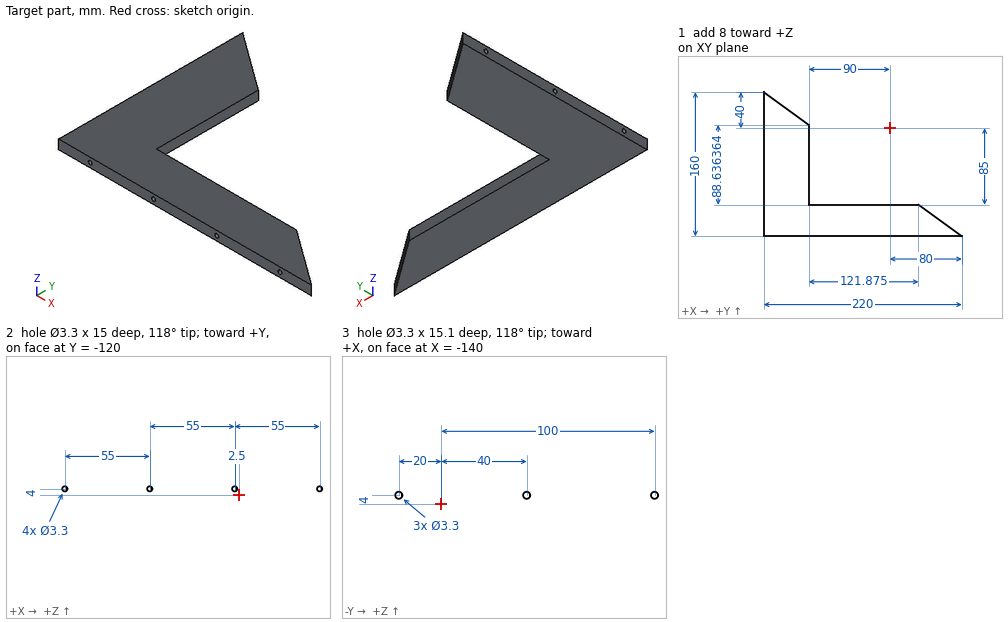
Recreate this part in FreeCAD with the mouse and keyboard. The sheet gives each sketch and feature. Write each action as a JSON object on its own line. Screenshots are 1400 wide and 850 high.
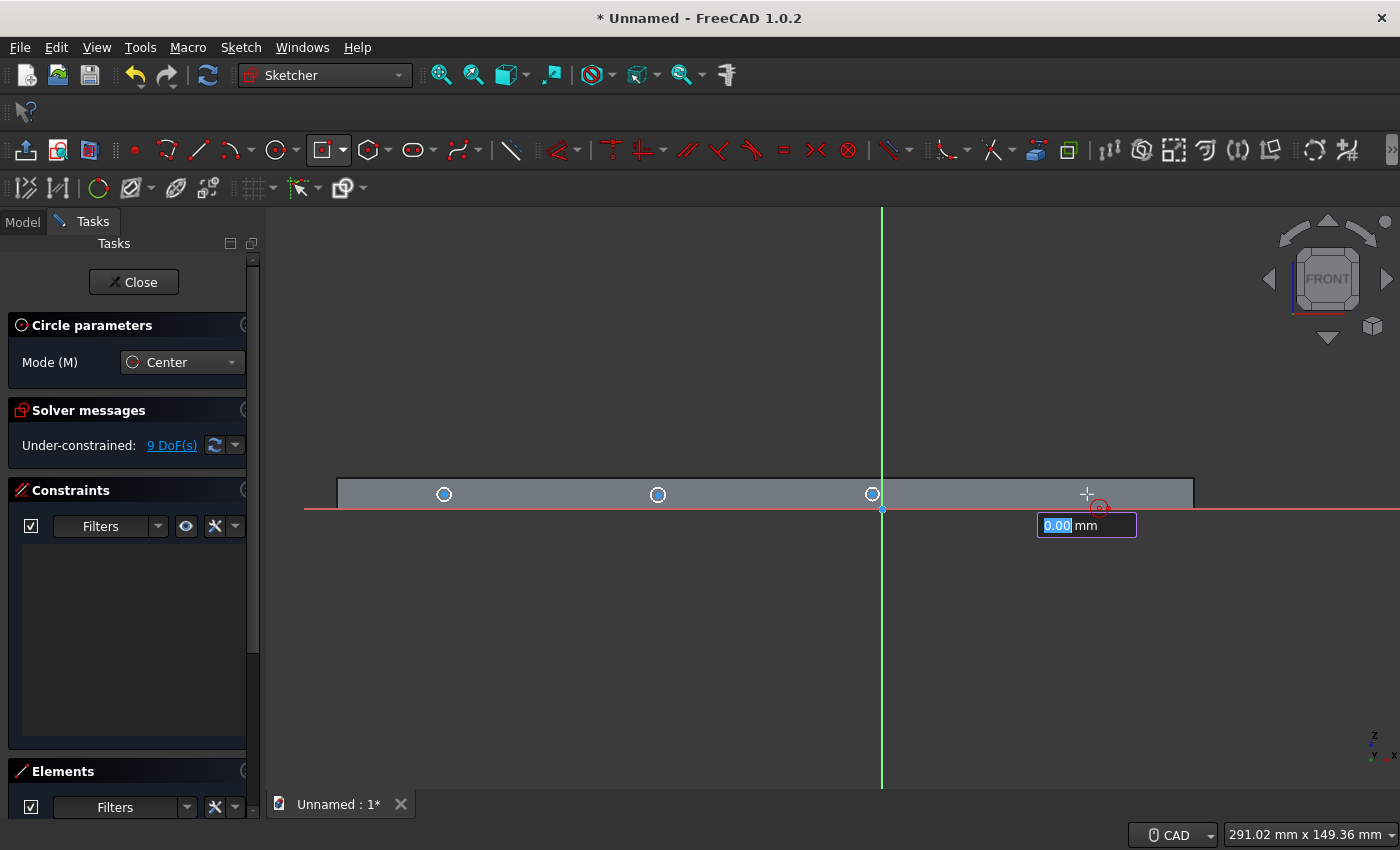
{"action": "scroll", "coordinate": [1091, 489], "scroll_direction": "up", "scroll_amount": 5}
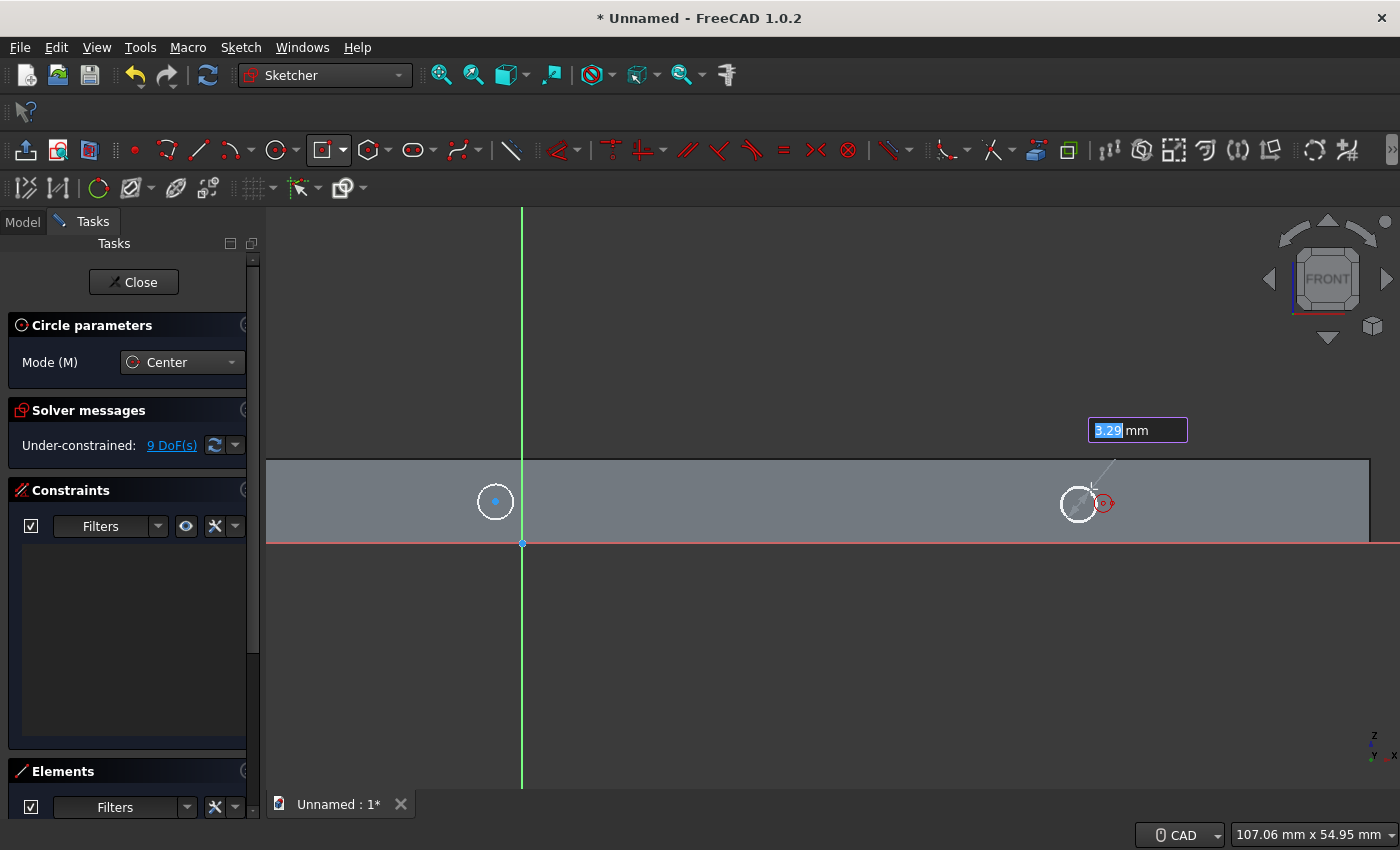
{"action": "left_click", "coordinate": [1091, 489]}
{"action": "key", "text": "Escape"}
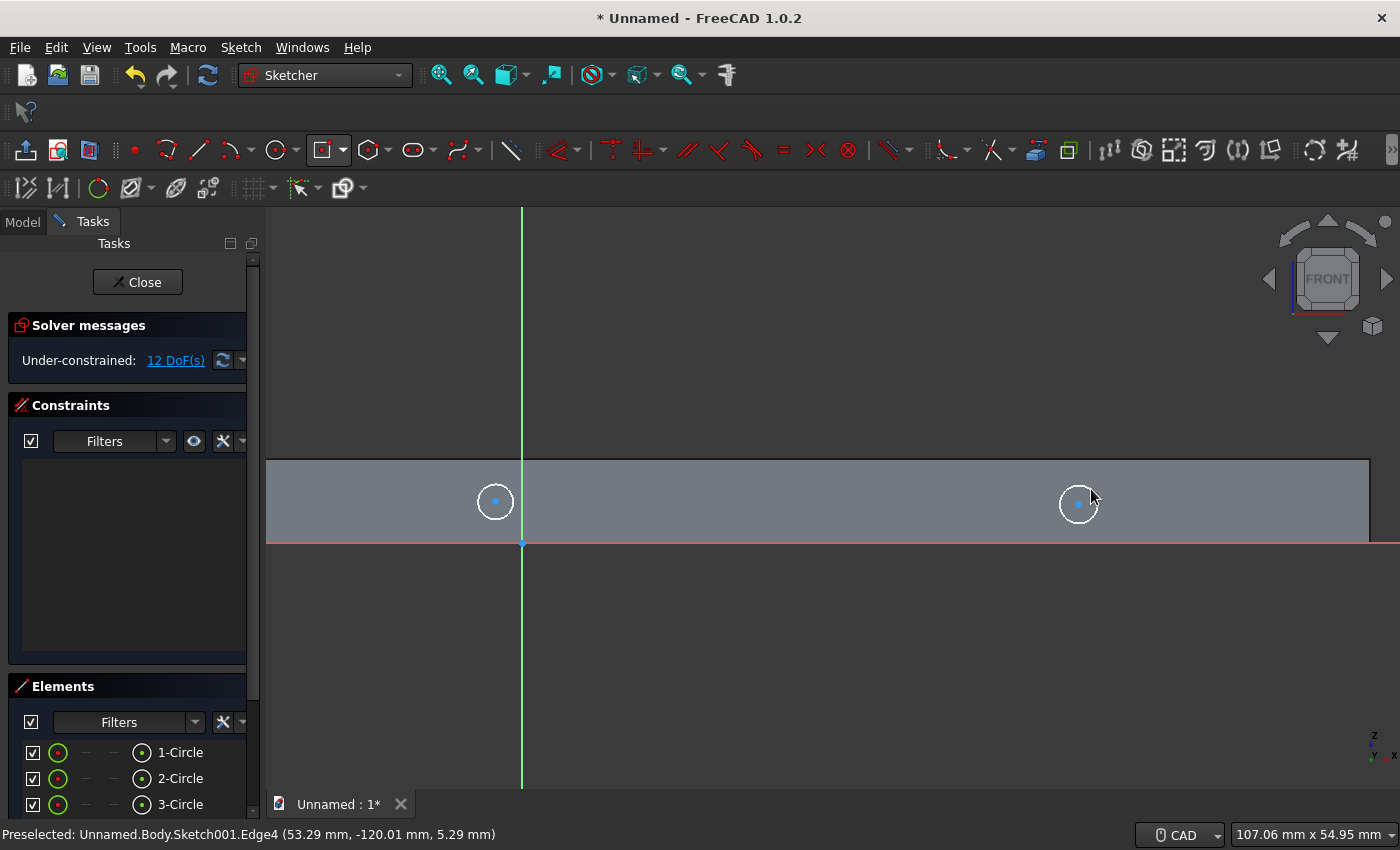
{"action": "scroll", "coordinate": [1090, 489], "scroll_direction": "down", "scroll_amount": 5}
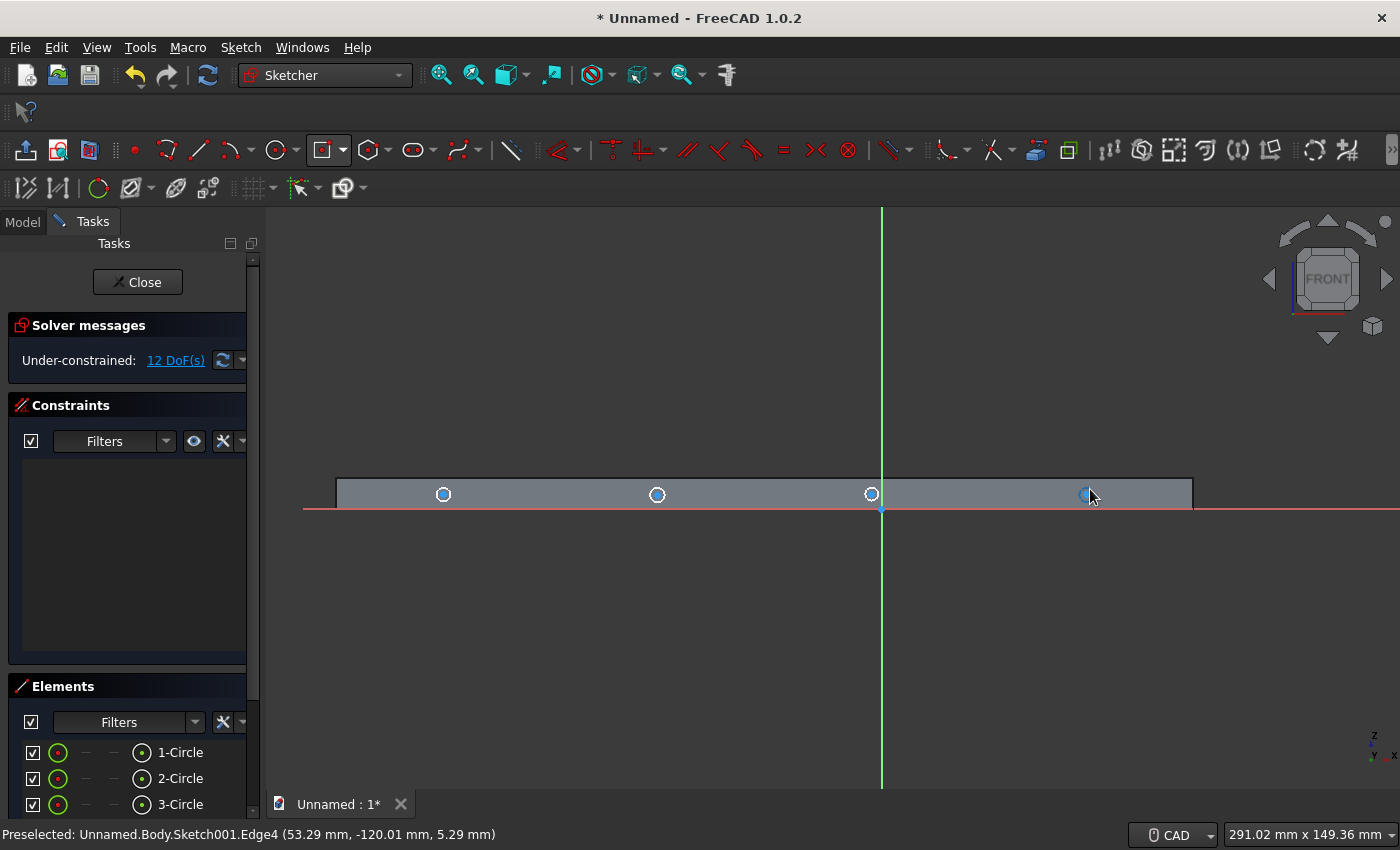
{"action": "scroll", "coordinate": [448, 490], "scroll_direction": "up", "scroll_amount": 4}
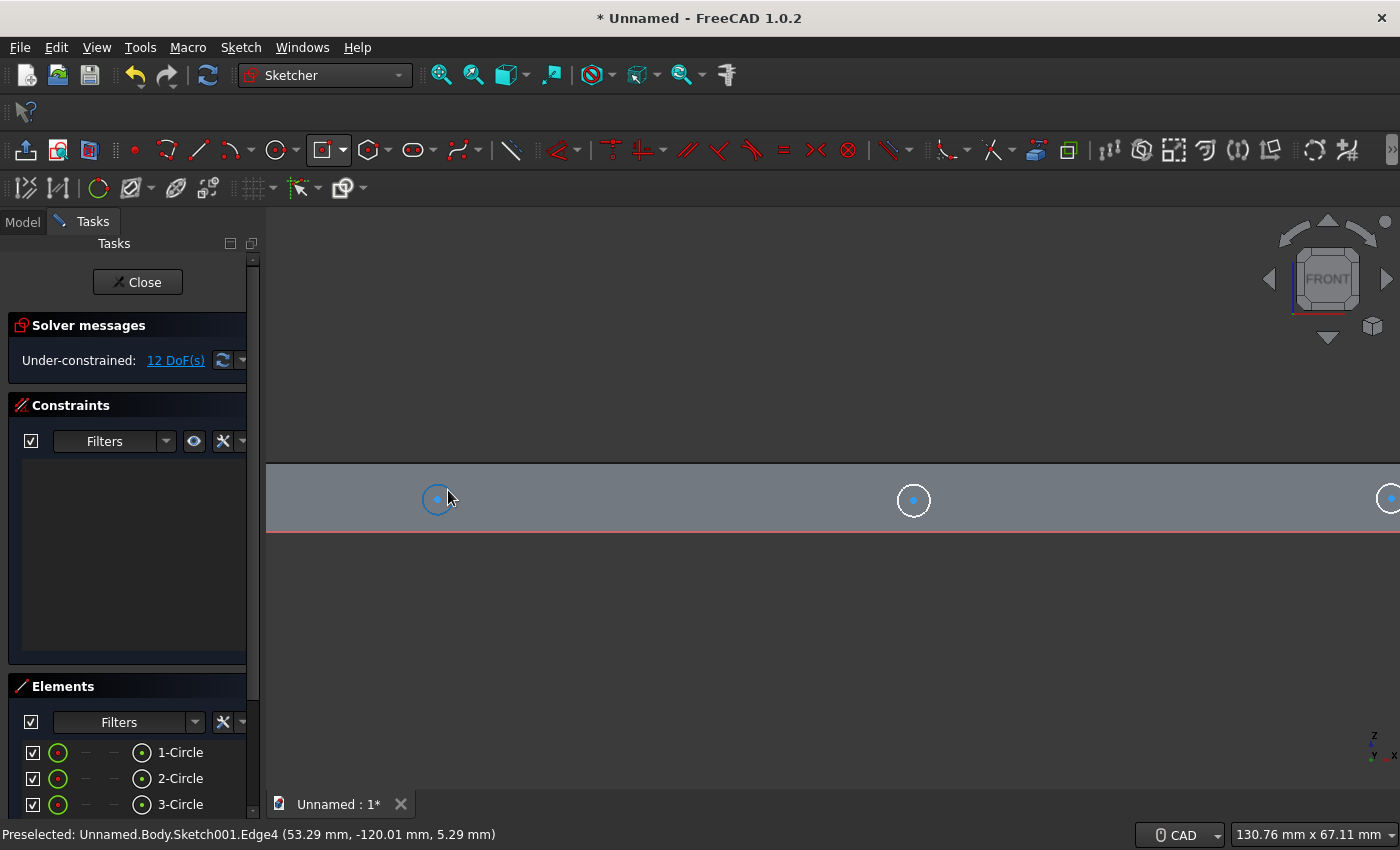
{"action": "left_click", "coordinate": [448, 489]}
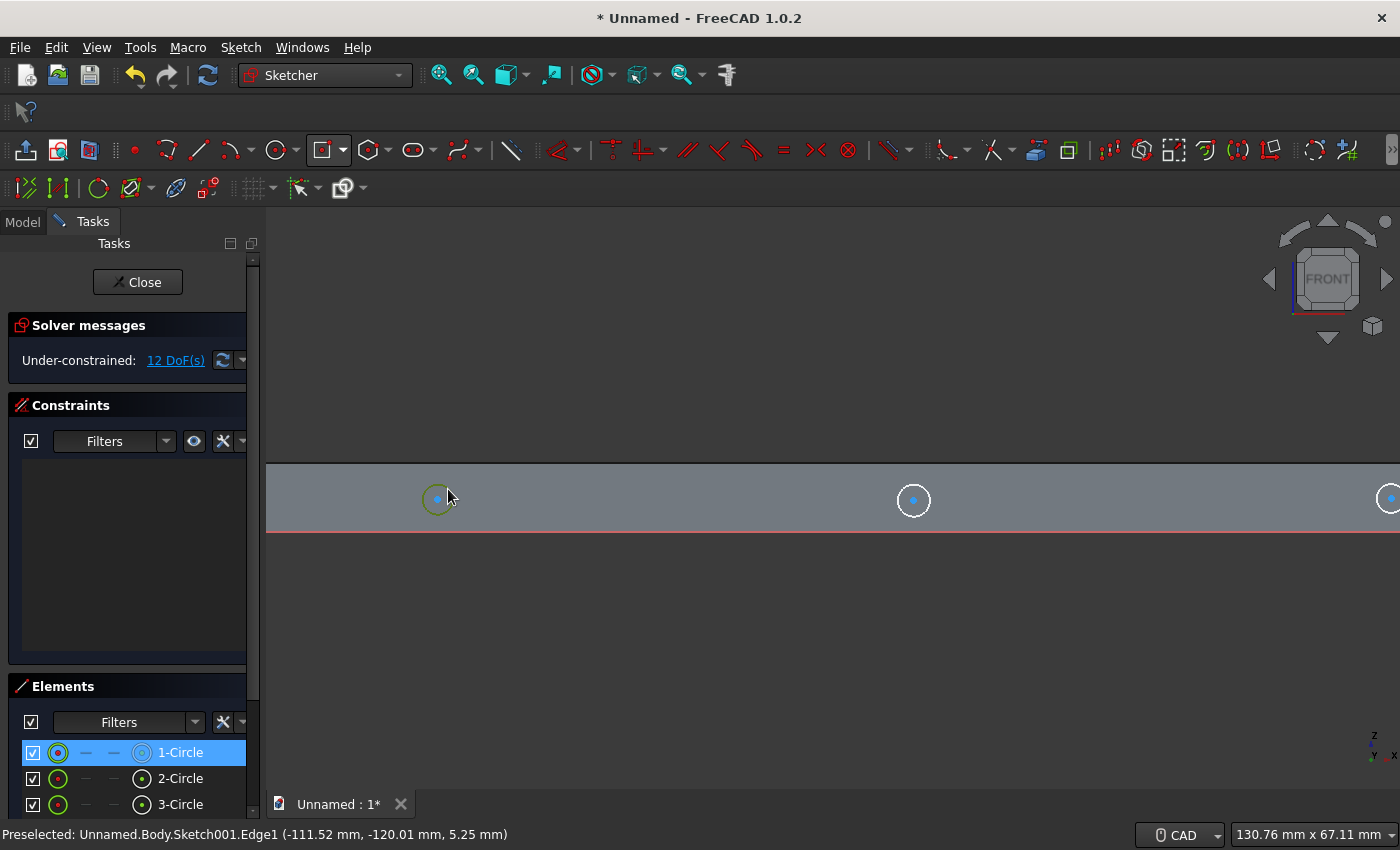
{"action": "left_click", "coordinate": [925, 489]}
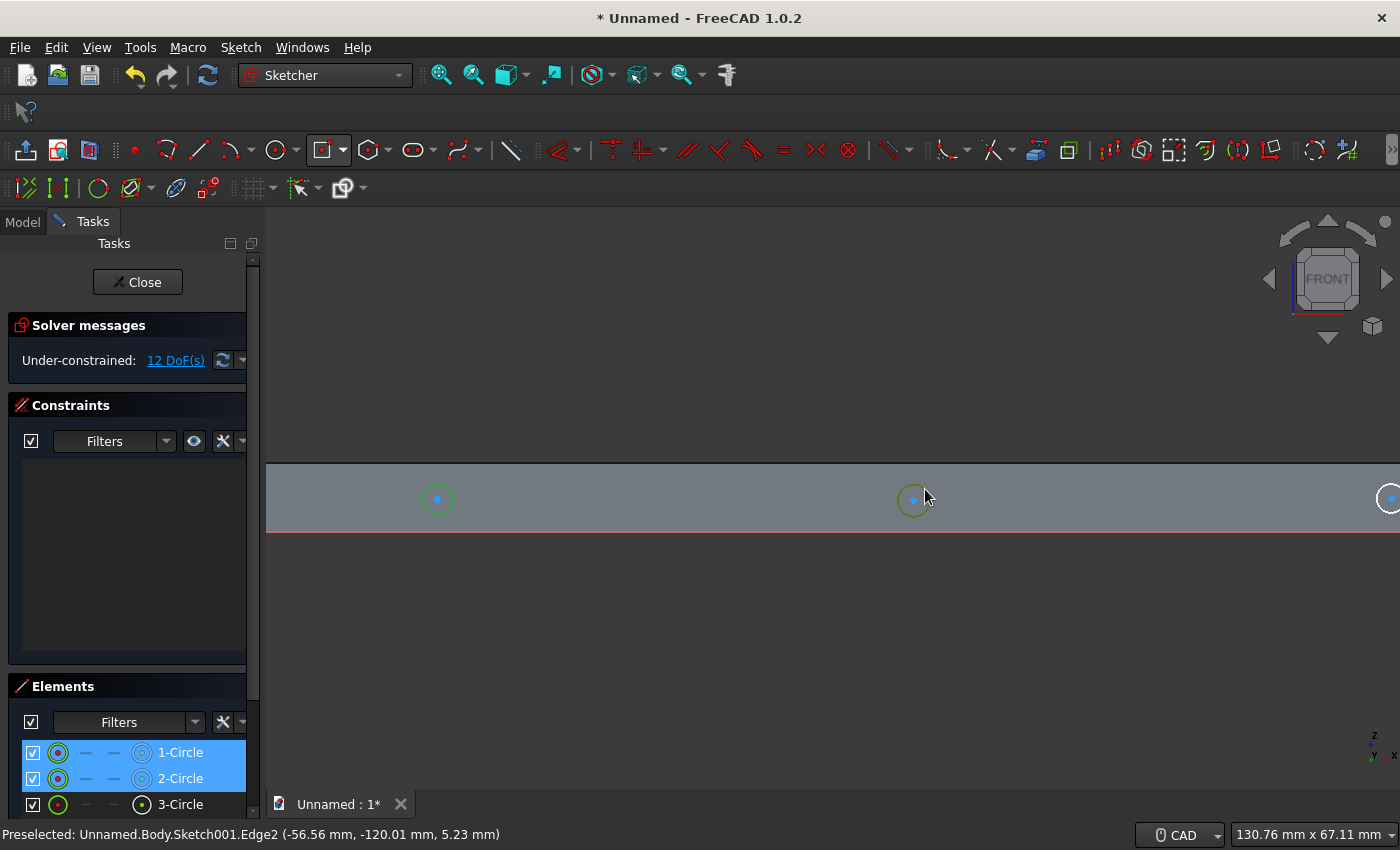
{"action": "scroll", "coordinate": [448, 490], "scroll_direction": "down", "scroll_amount": 4}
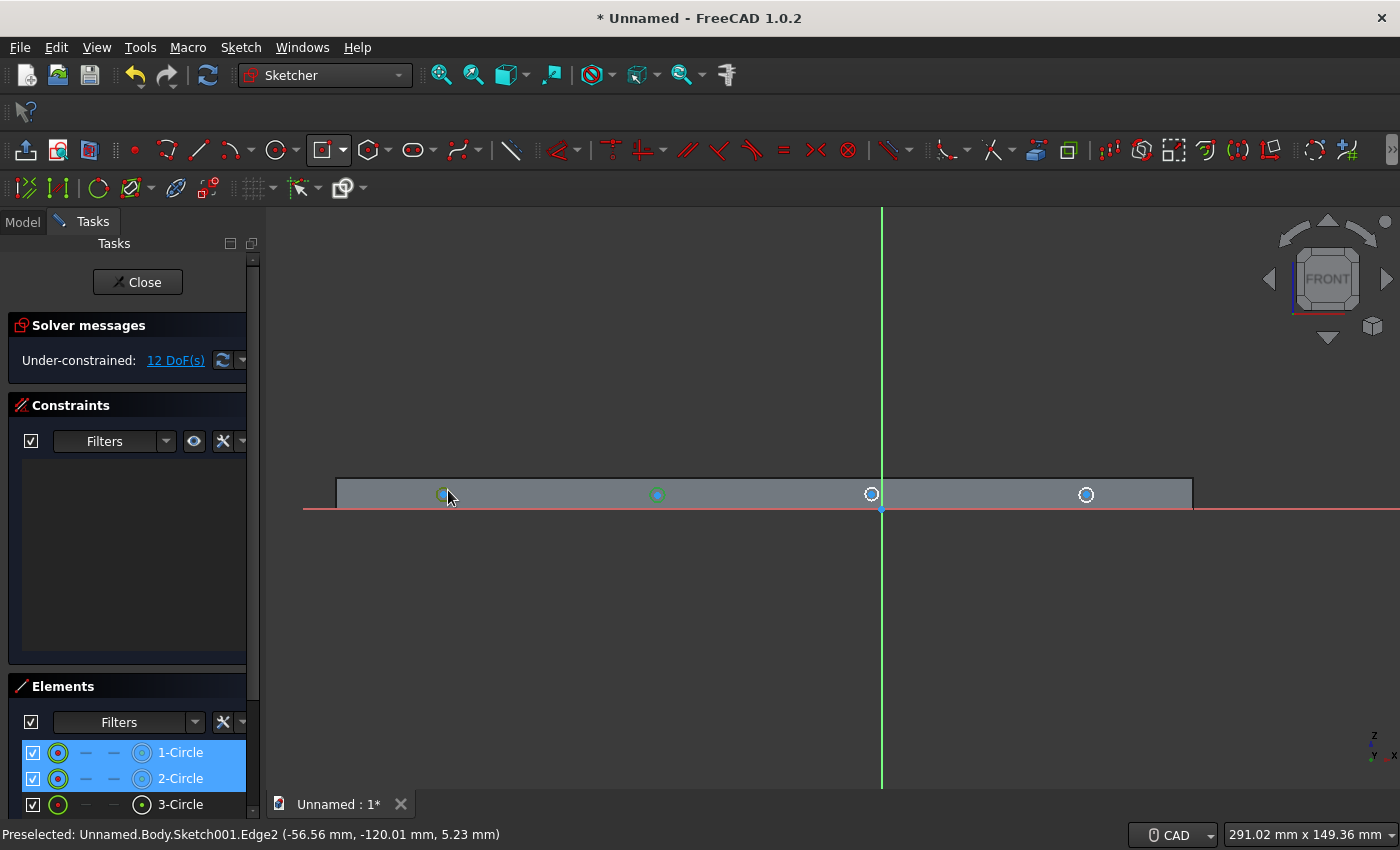
{"action": "scroll", "coordinate": [876, 490], "scroll_direction": "up", "scroll_amount": 5}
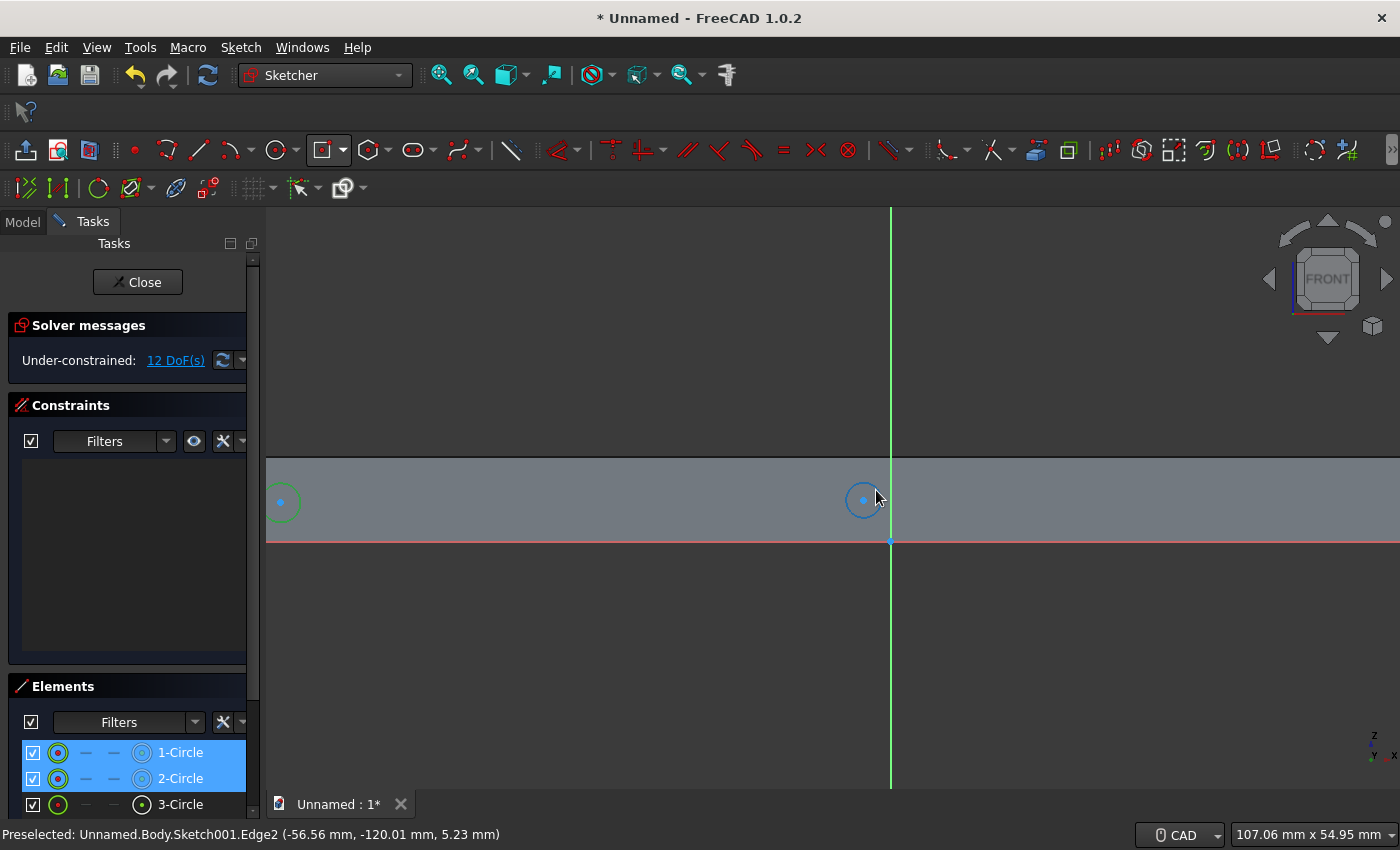
{"action": "left_click", "coordinate": [876, 488]}